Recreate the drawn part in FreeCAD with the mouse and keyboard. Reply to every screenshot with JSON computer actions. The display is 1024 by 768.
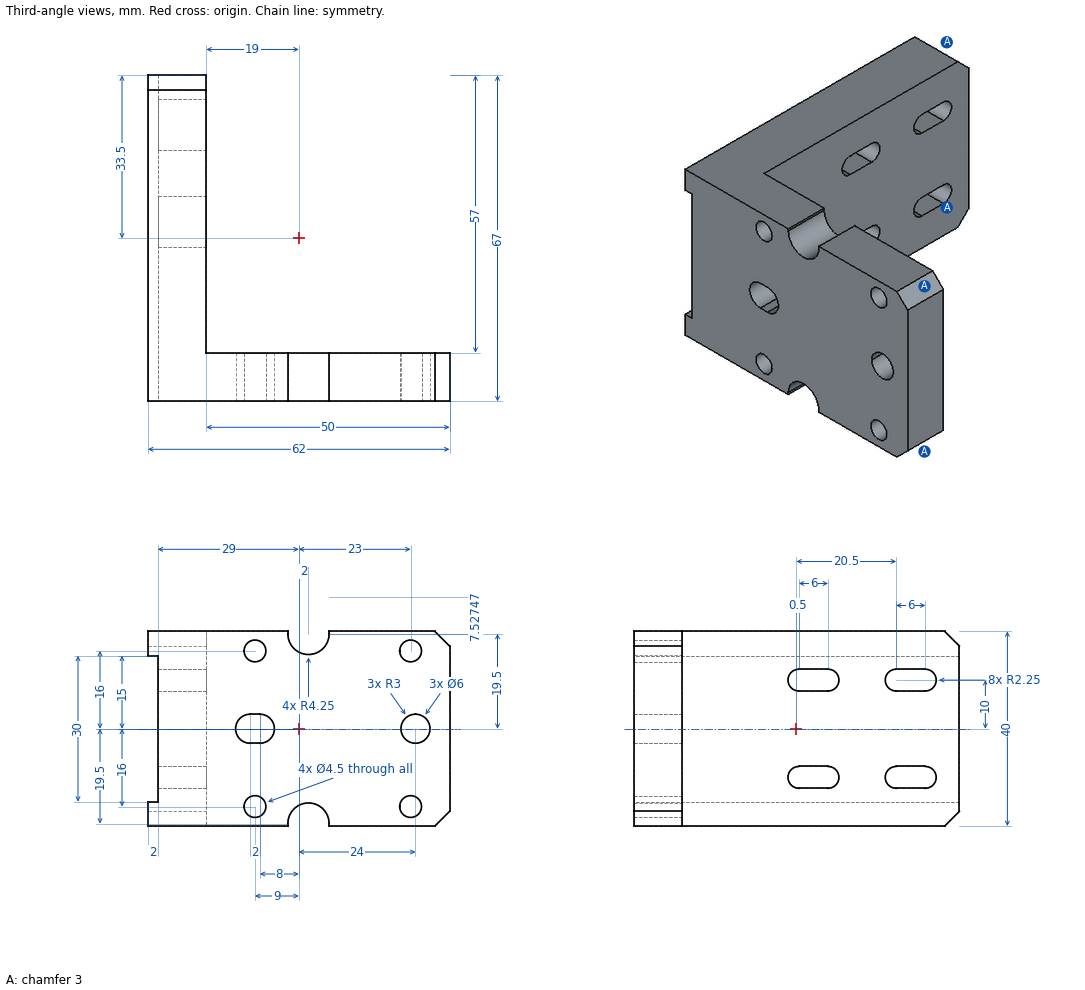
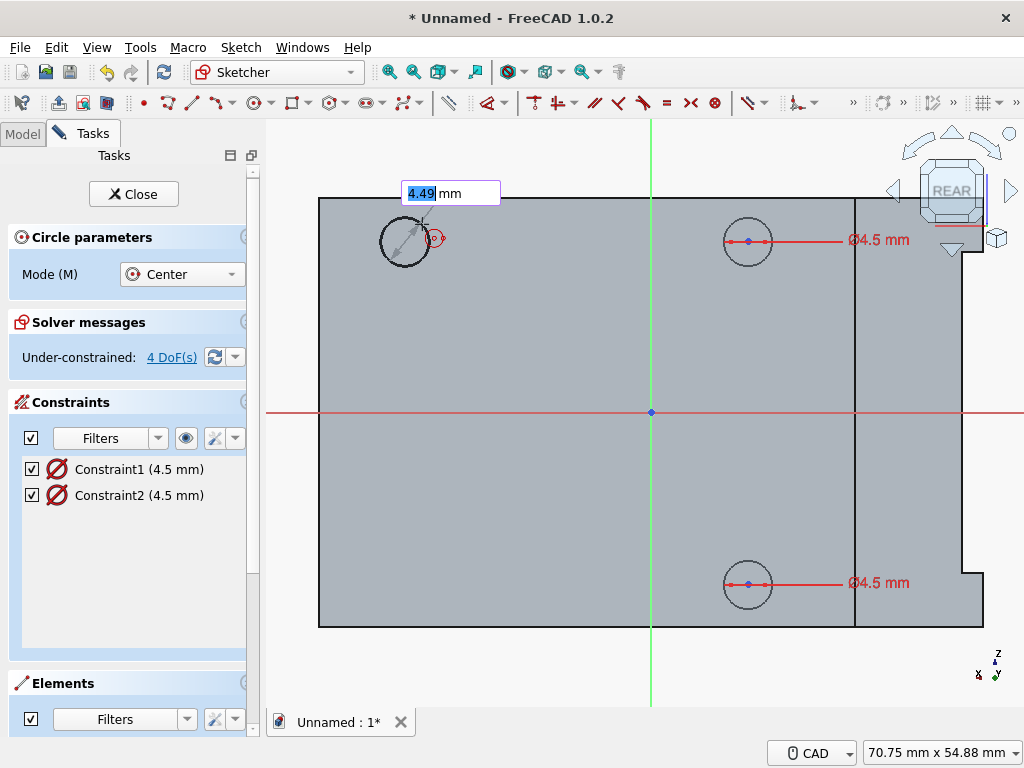
{"action": "type", "text": "4.5"}
{"action": "key", "text": "Return"}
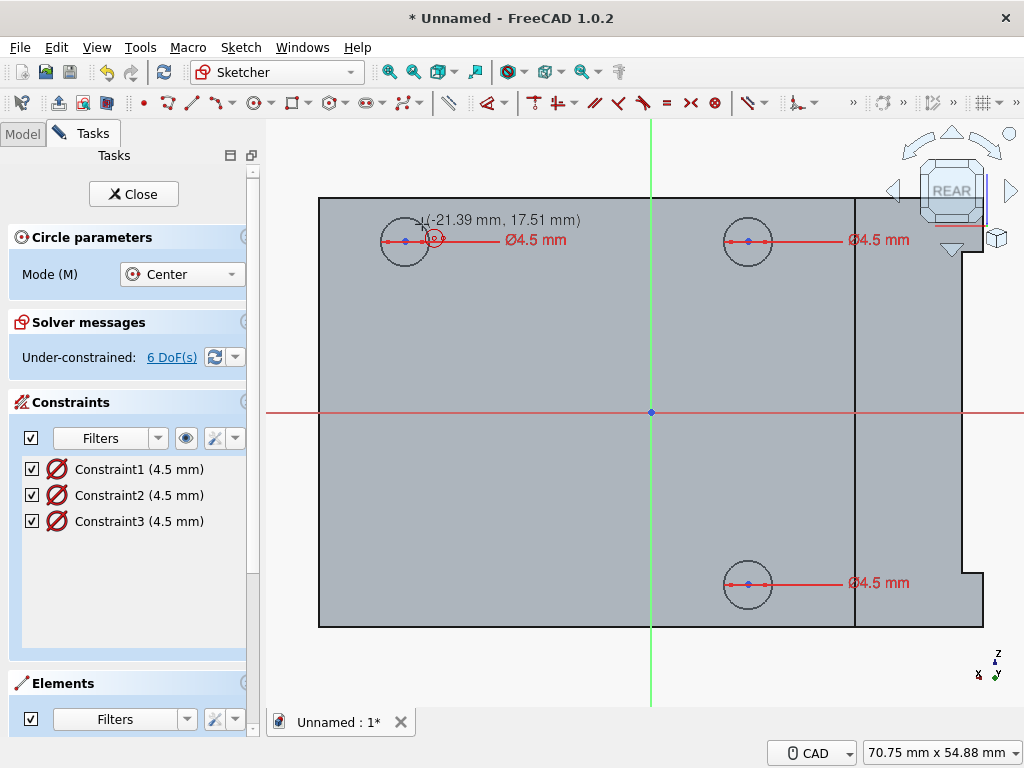
{"action": "left_click", "coordinate": [405, 584]}
{"action": "mouse_move", "coordinate": [422, 567]}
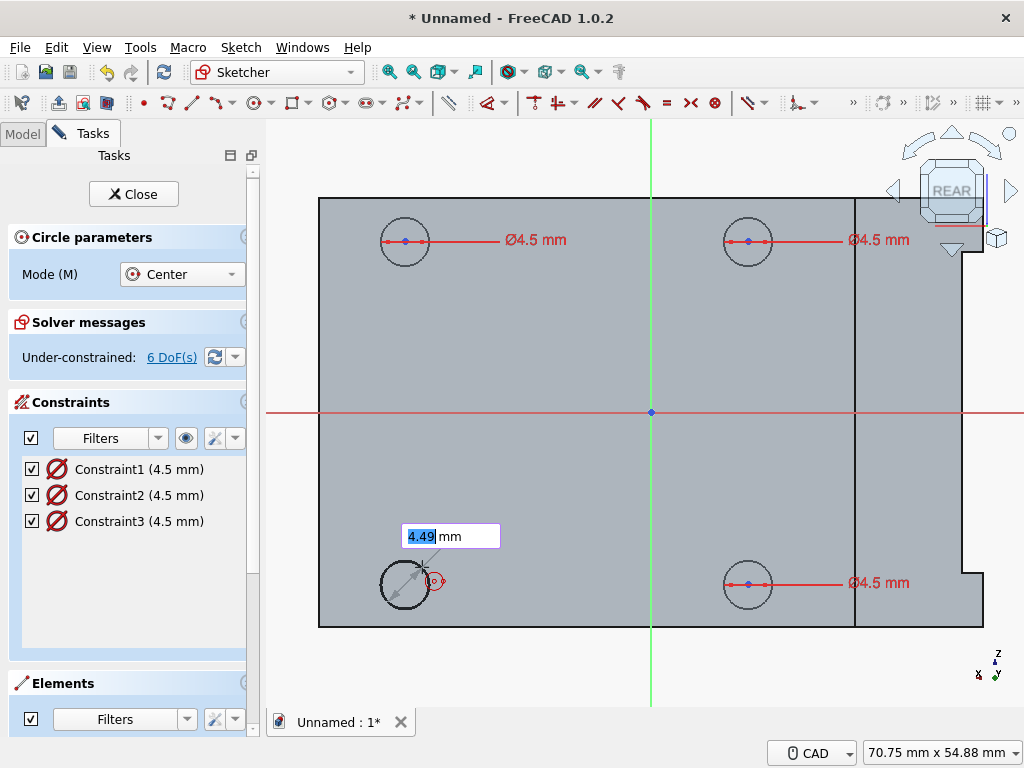
{"action": "type", "text": "4.5"}
{"action": "key", "text": "Return"}
{"action": "key", "text": "Escape"}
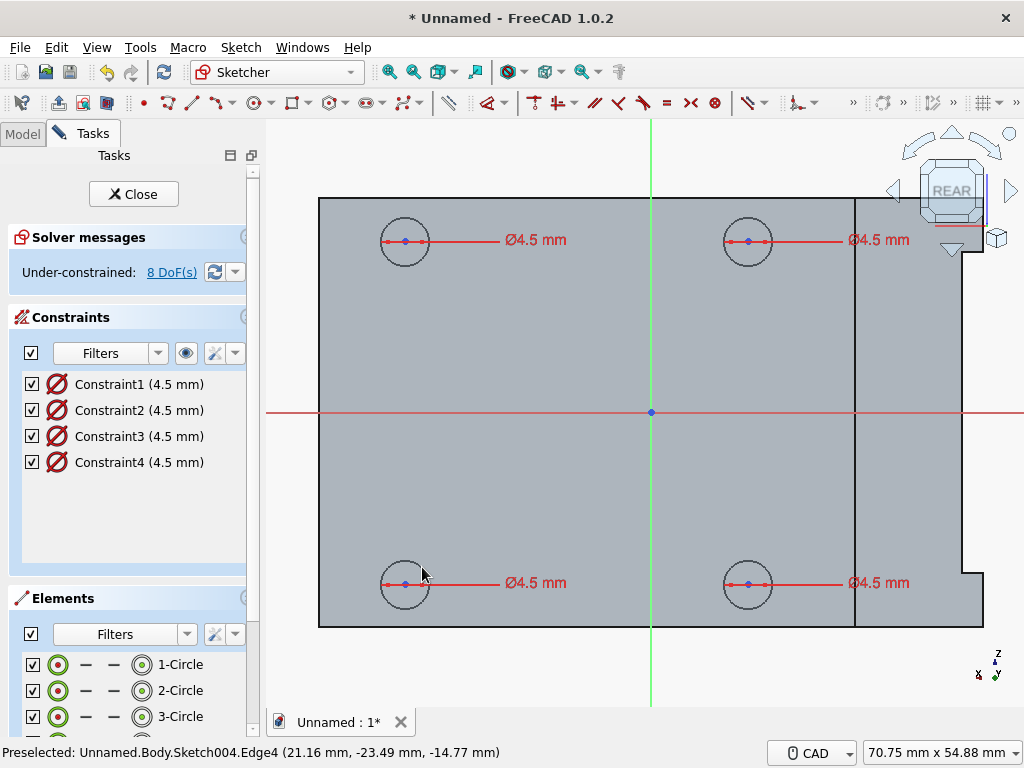
{"action": "left_click", "coordinate": [748, 585]}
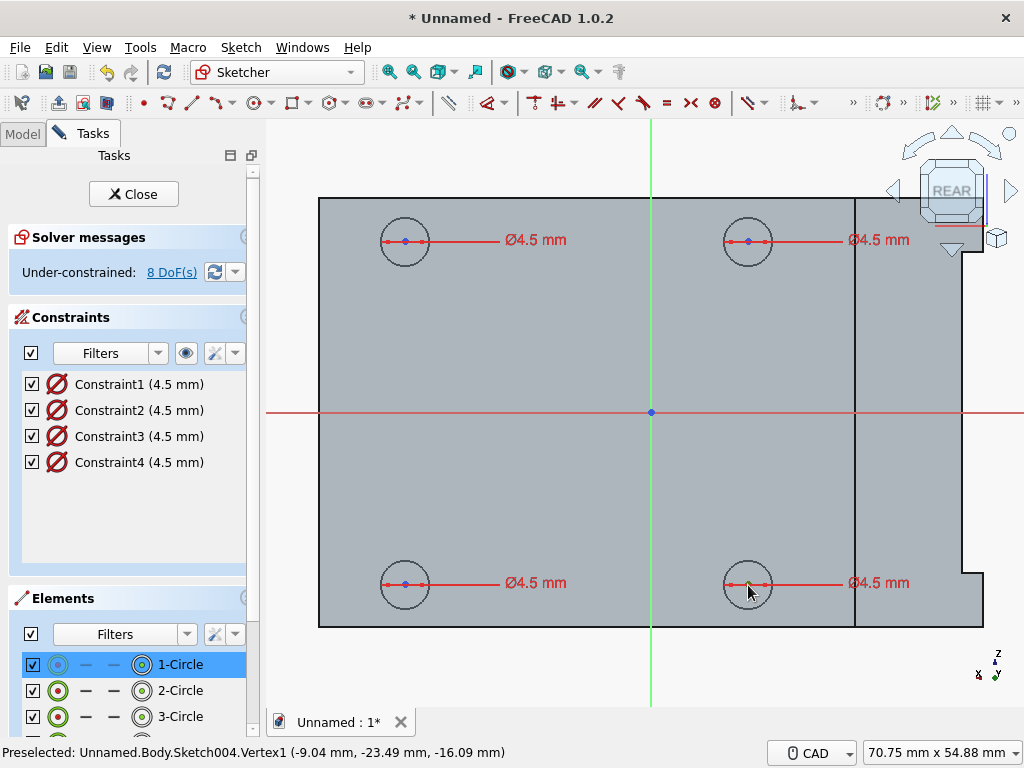
{"action": "left_click", "coordinate": [748, 242]}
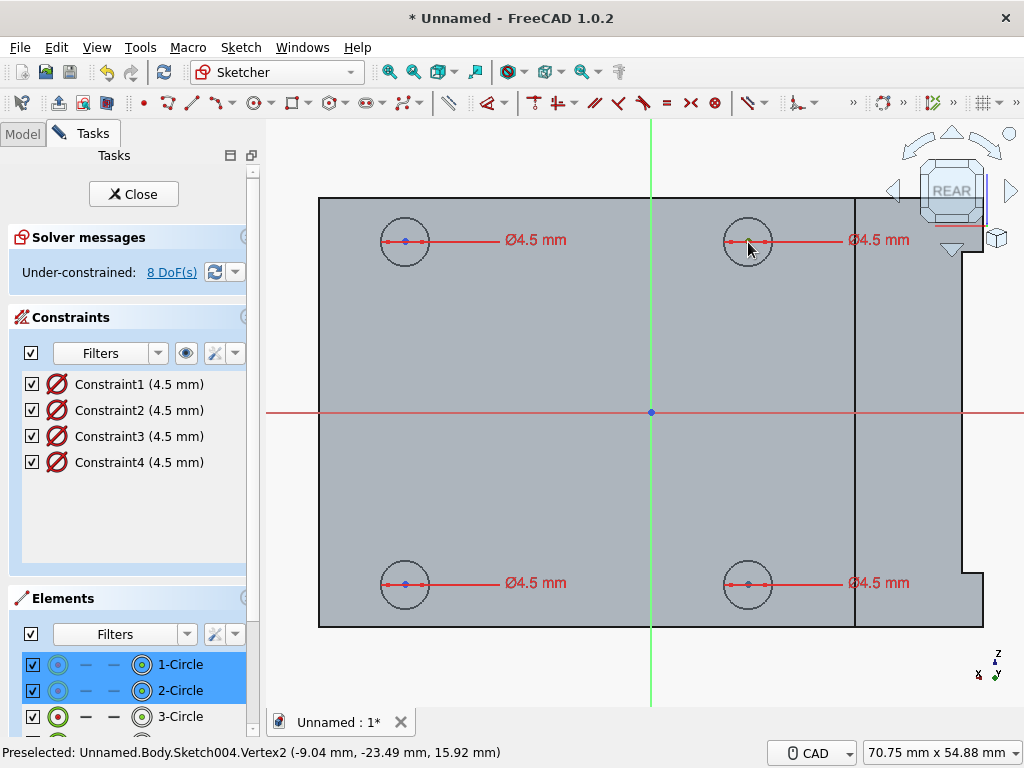
{"action": "left_click", "coordinate": [576, 104]}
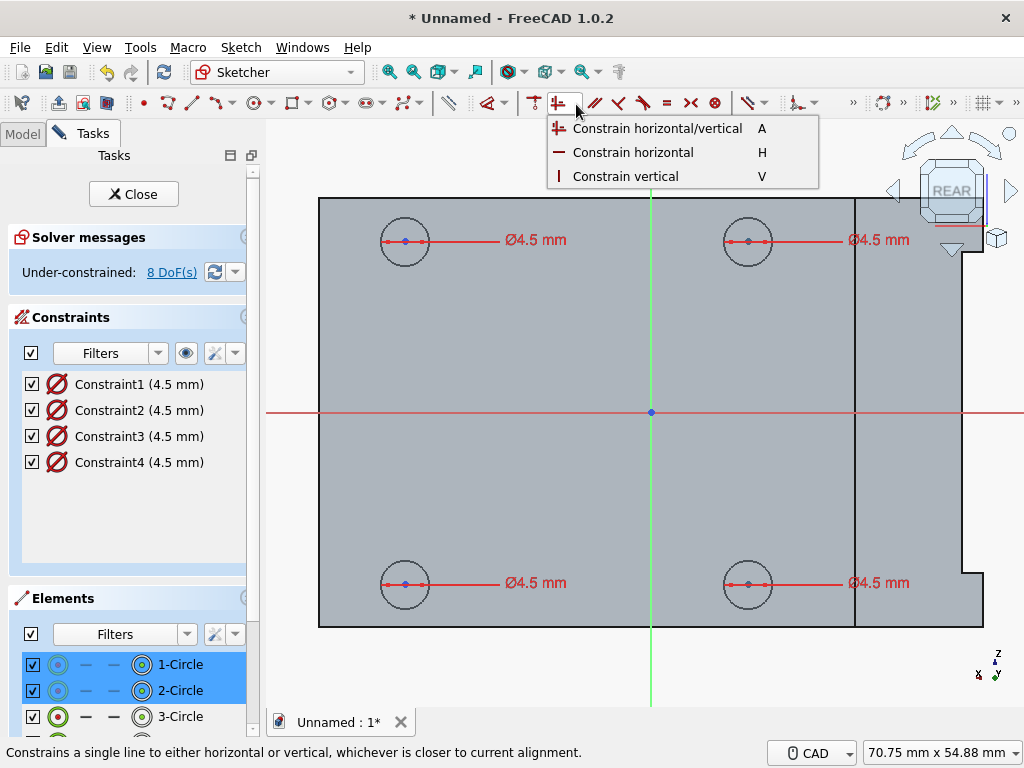
{"action": "left_click", "coordinate": [683, 176]}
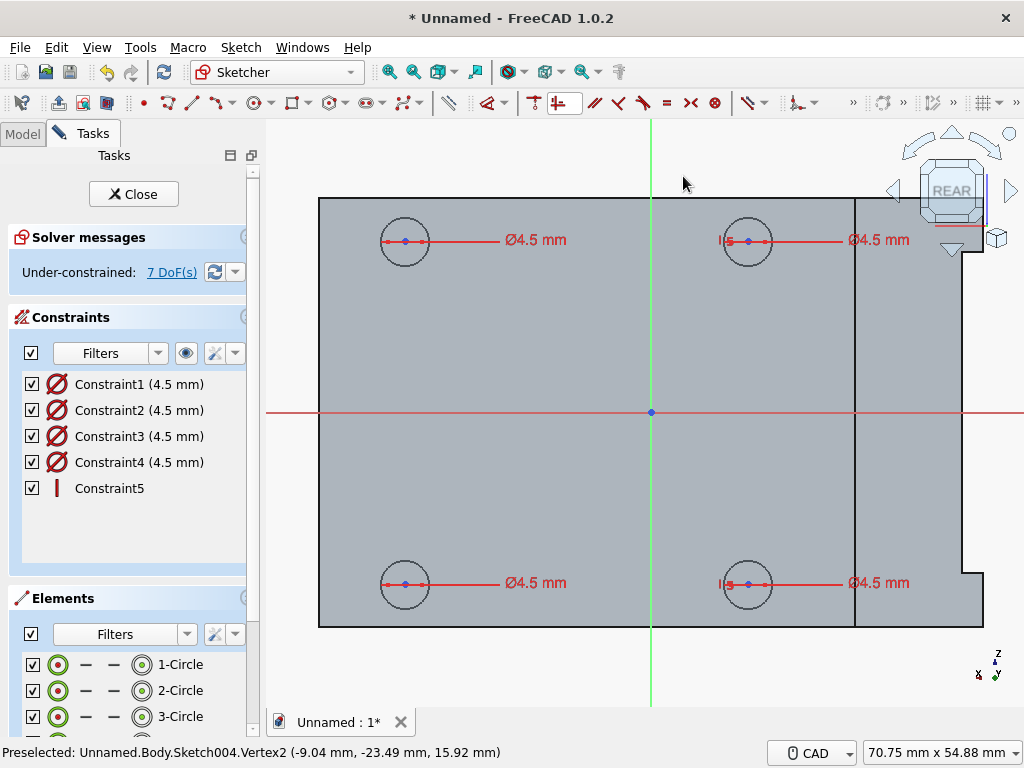
{"action": "left_click", "coordinate": [748, 242]}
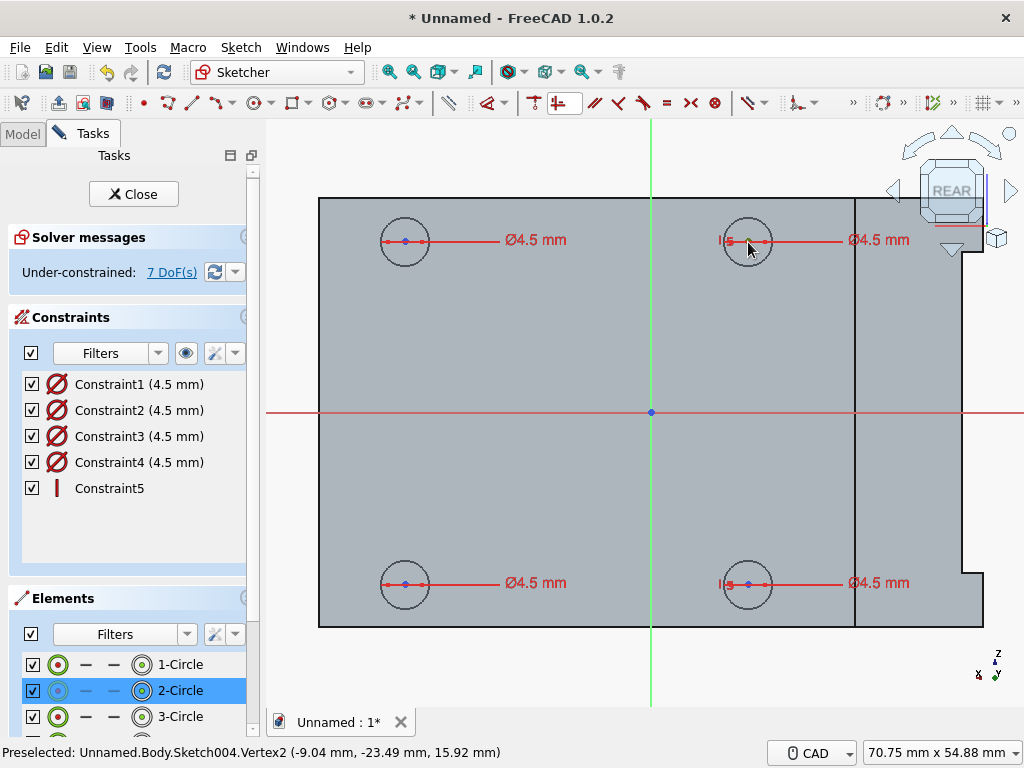
{"action": "left_click", "coordinate": [405, 242]}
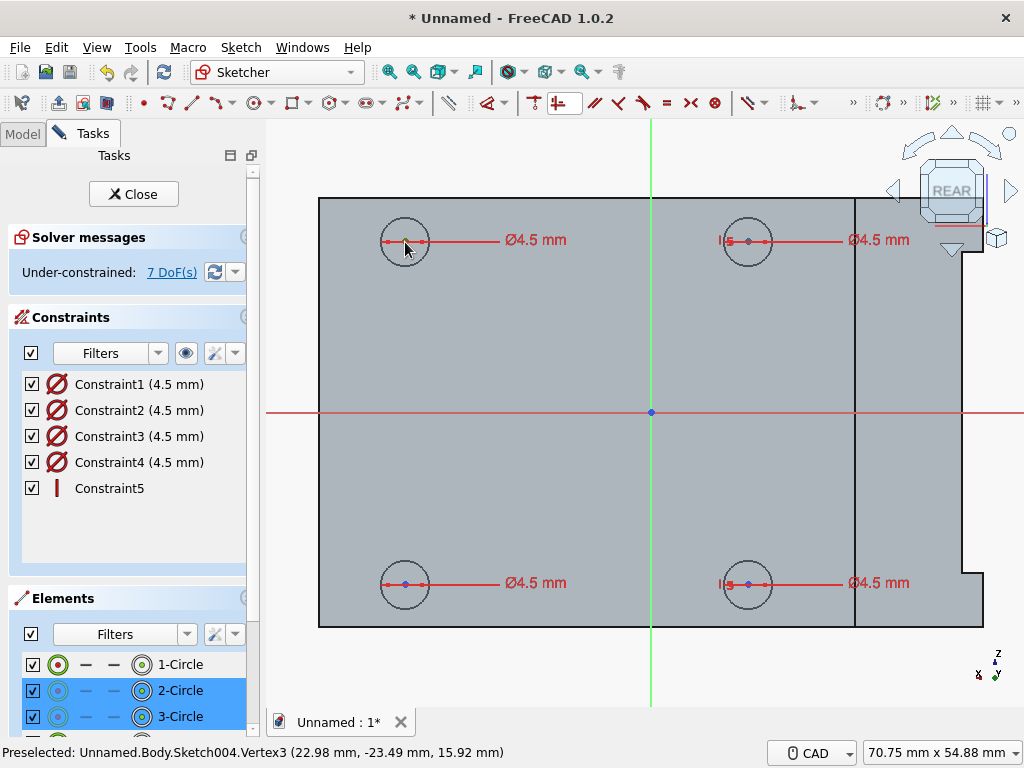
{"action": "key", "text": "h"}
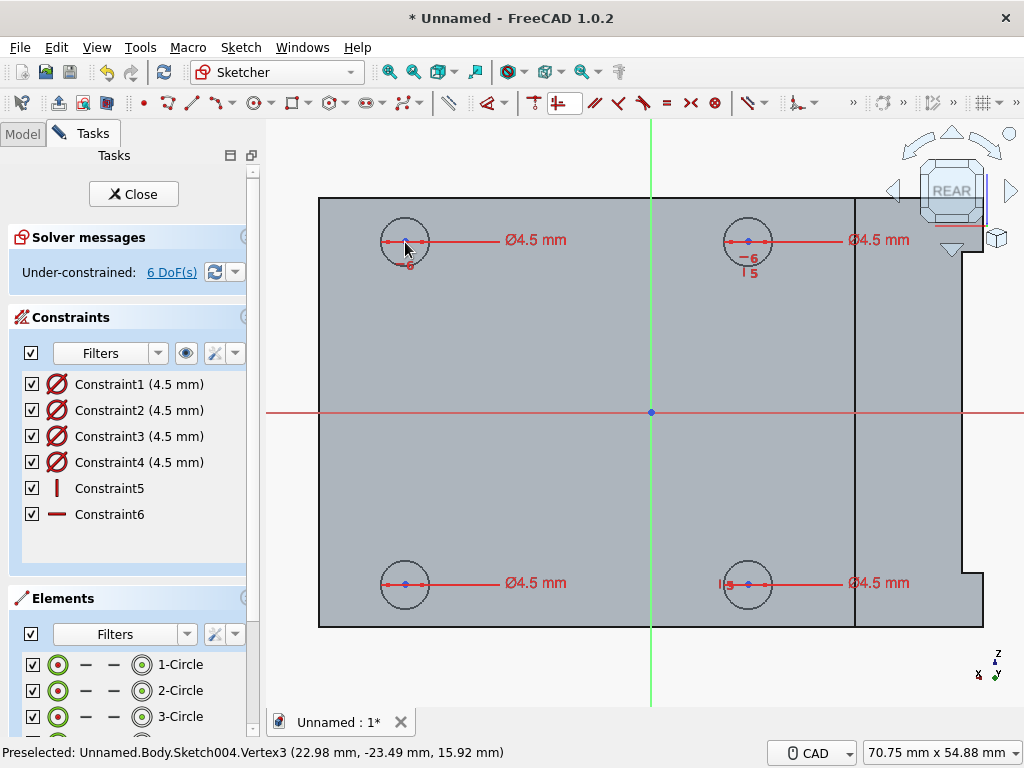
{"action": "left_click", "coordinate": [405, 242]}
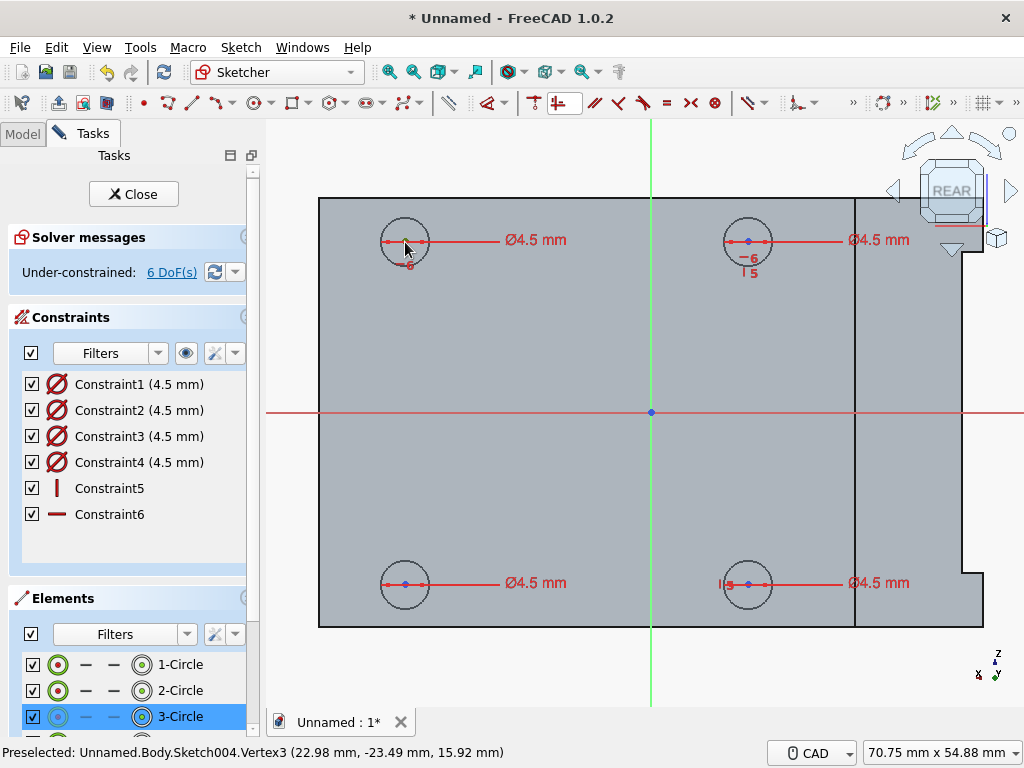
{"action": "left_click", "coordinate": [405, 585]}